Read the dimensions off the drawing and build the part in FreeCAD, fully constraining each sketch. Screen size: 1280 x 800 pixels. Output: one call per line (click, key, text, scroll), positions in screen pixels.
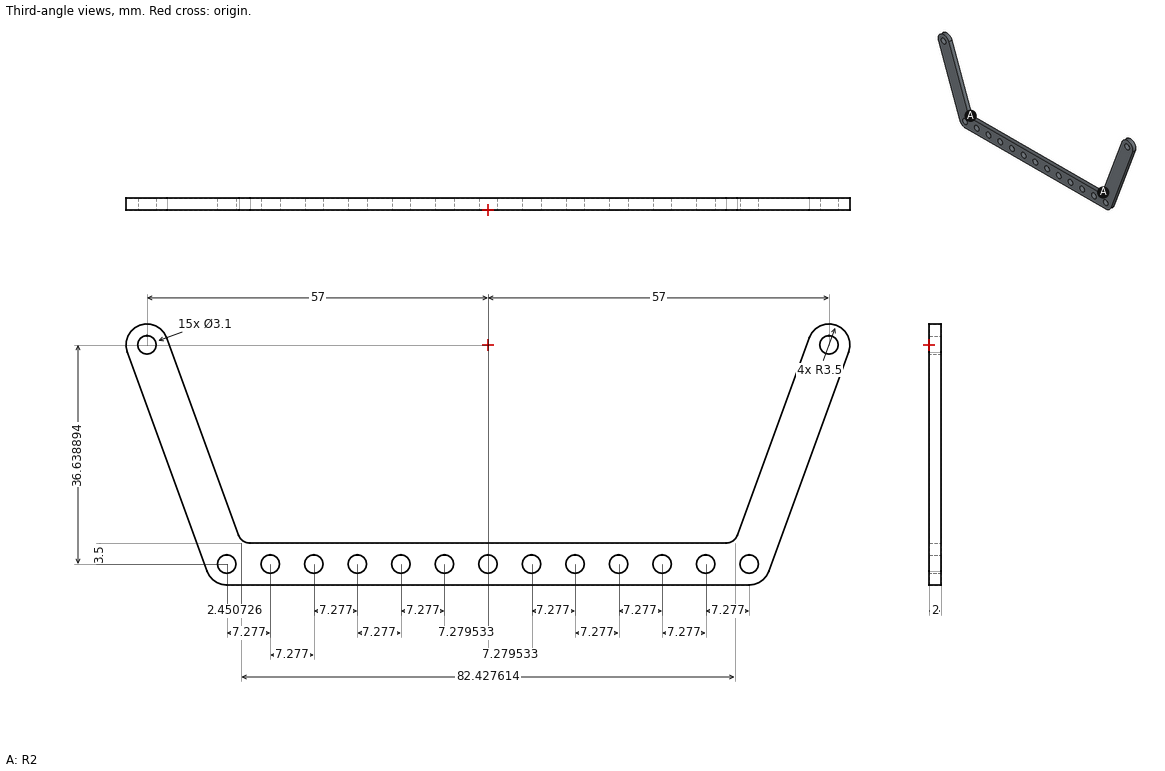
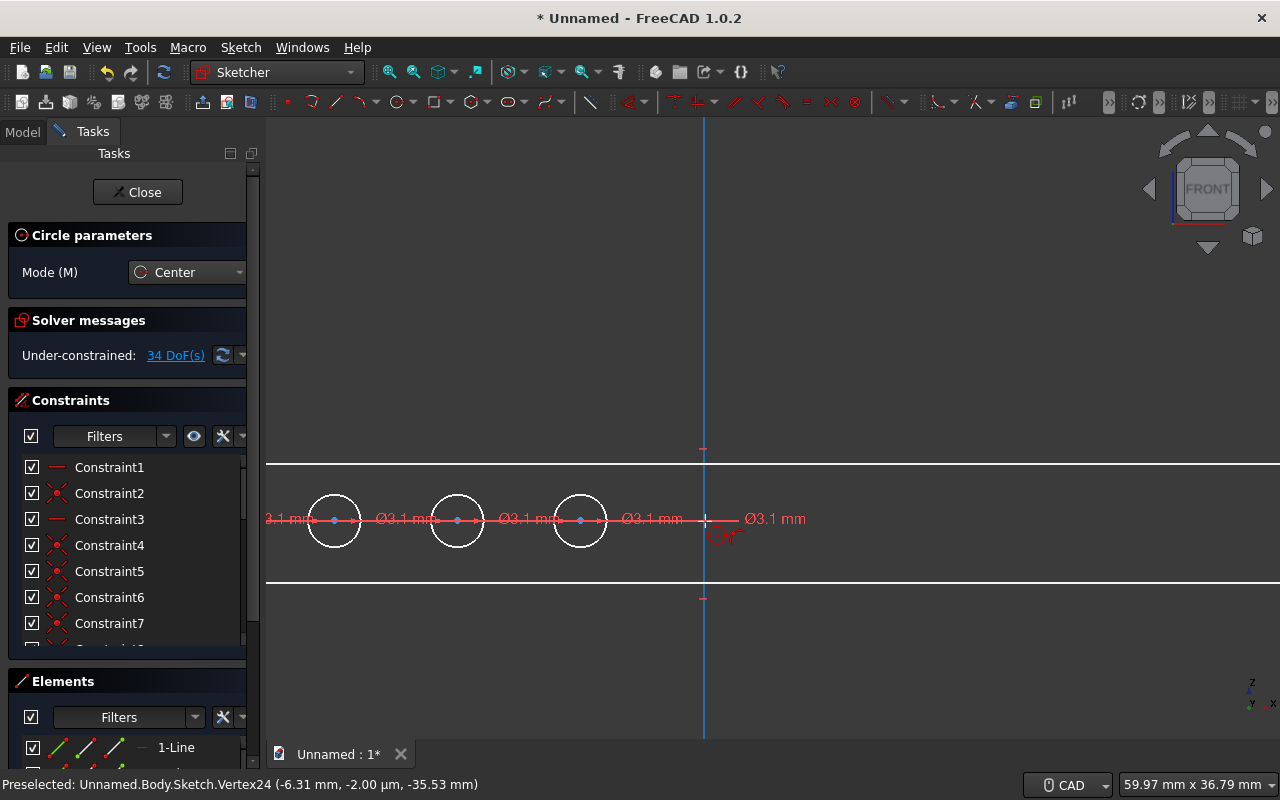
click(704, 520)
move(722, 501)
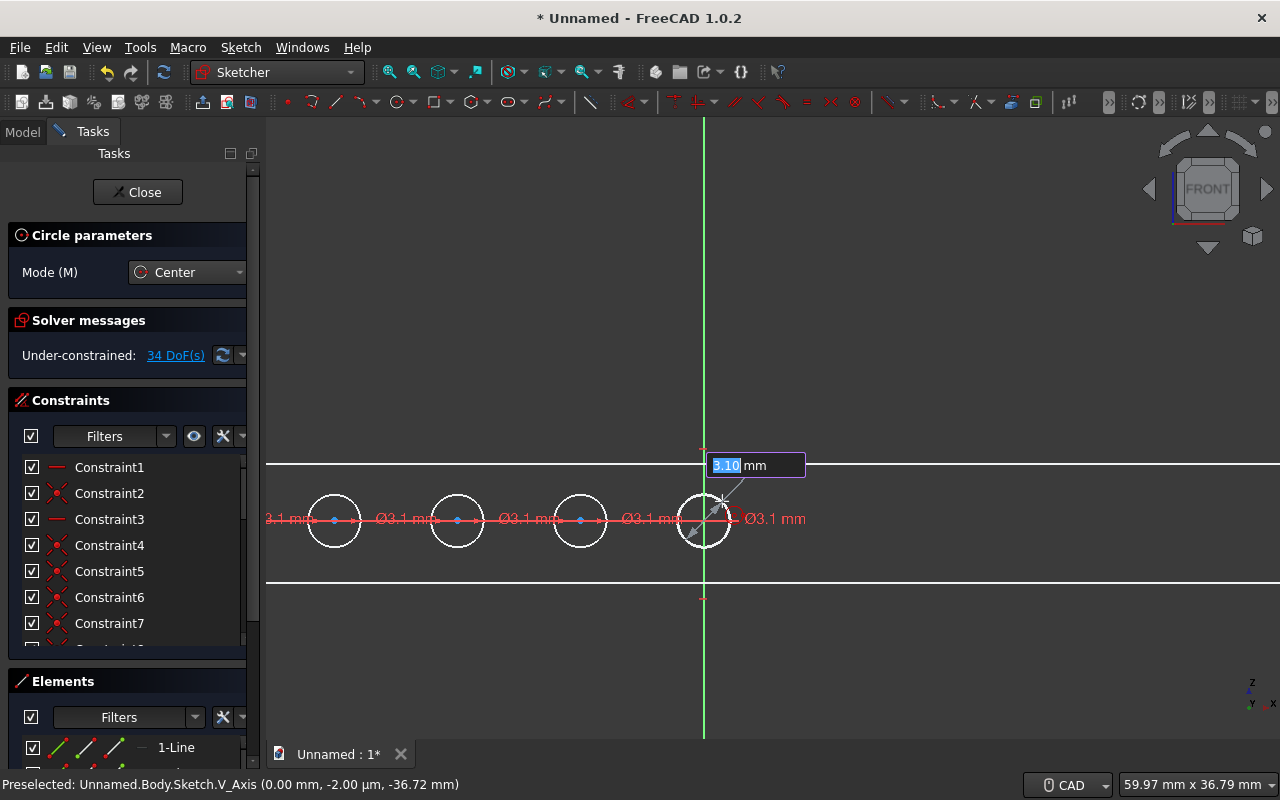
text(3.1)
key(Return)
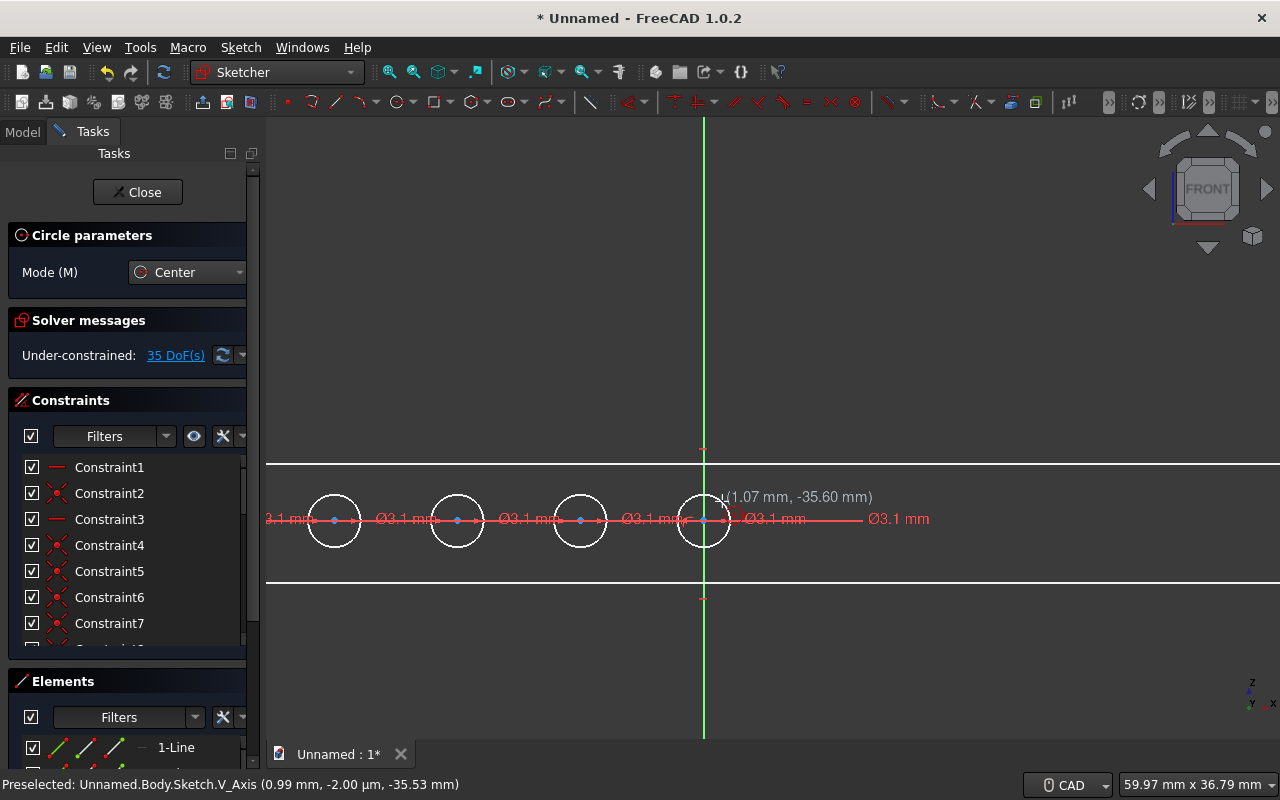
click(827, 520)
move(846, 501)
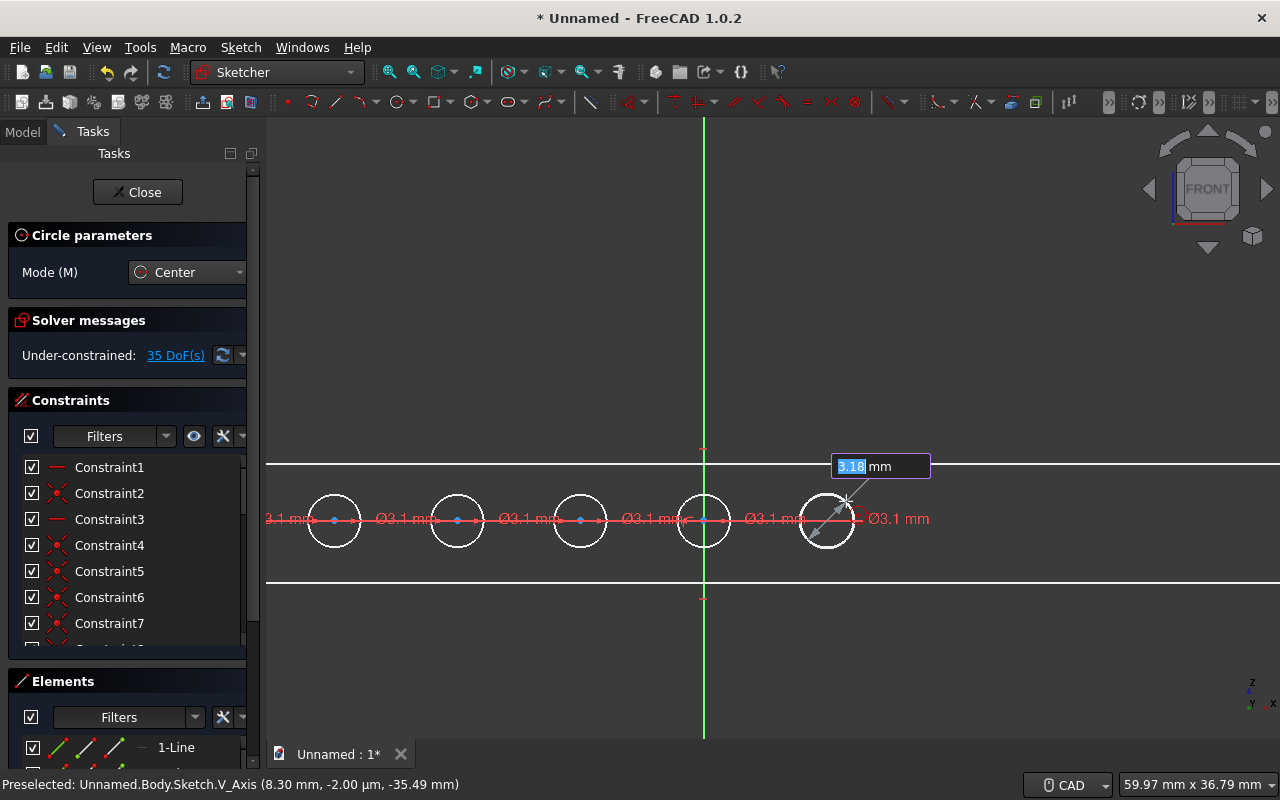
text(3.1)
key(Return)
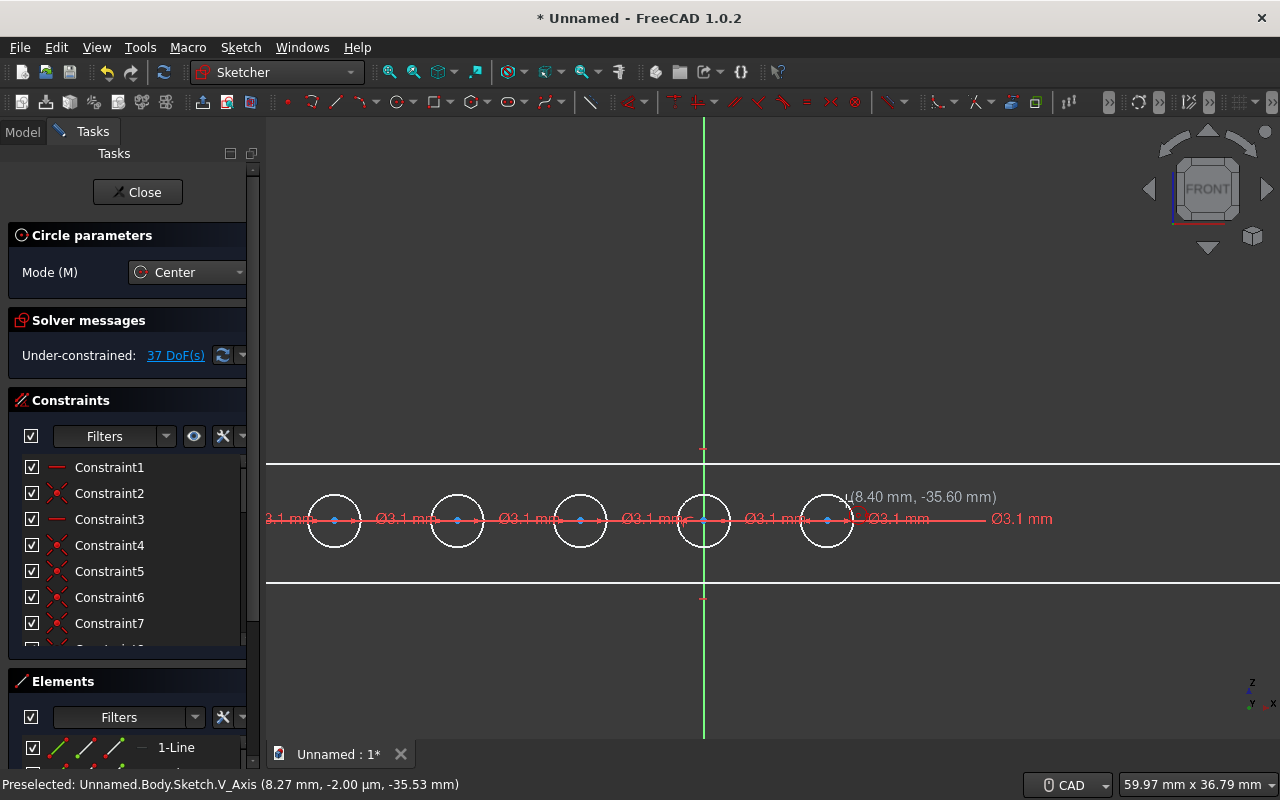
click(950, 520)
move(969, 501)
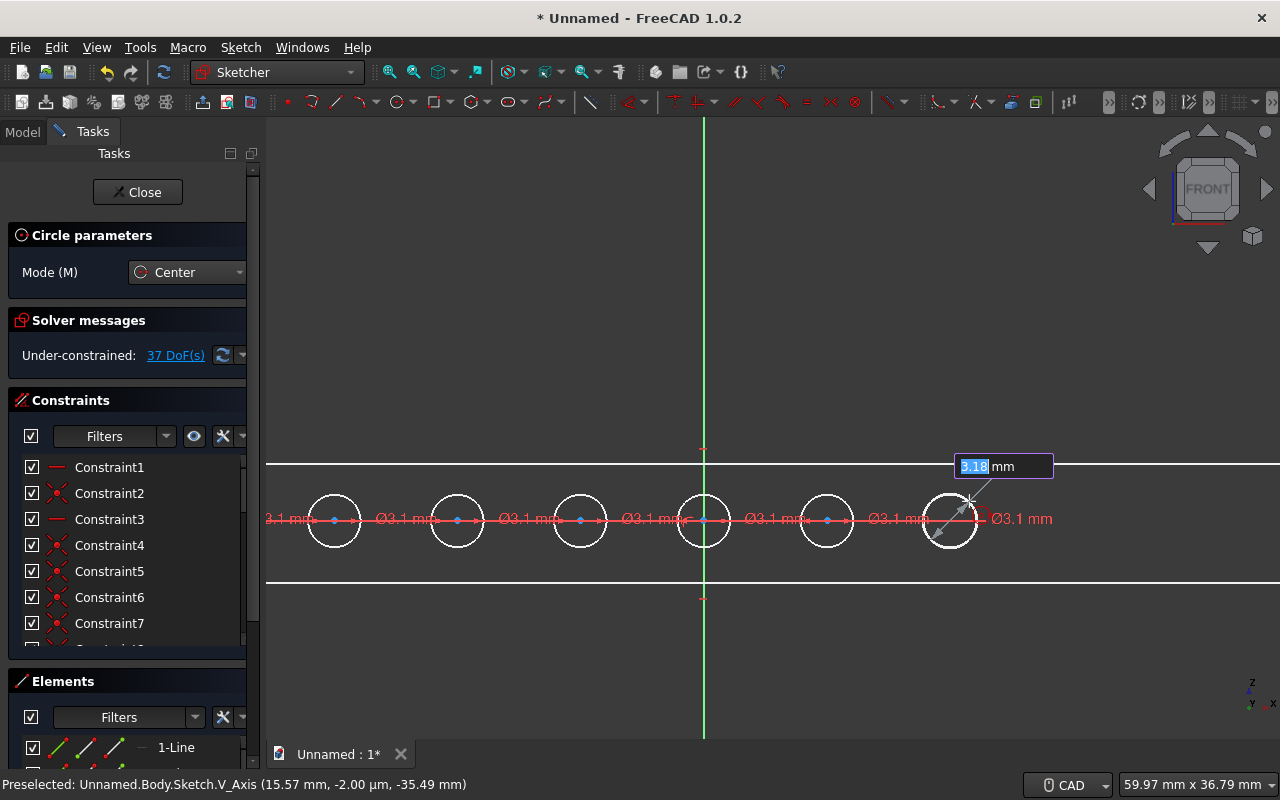
text(3.1)
key(Return)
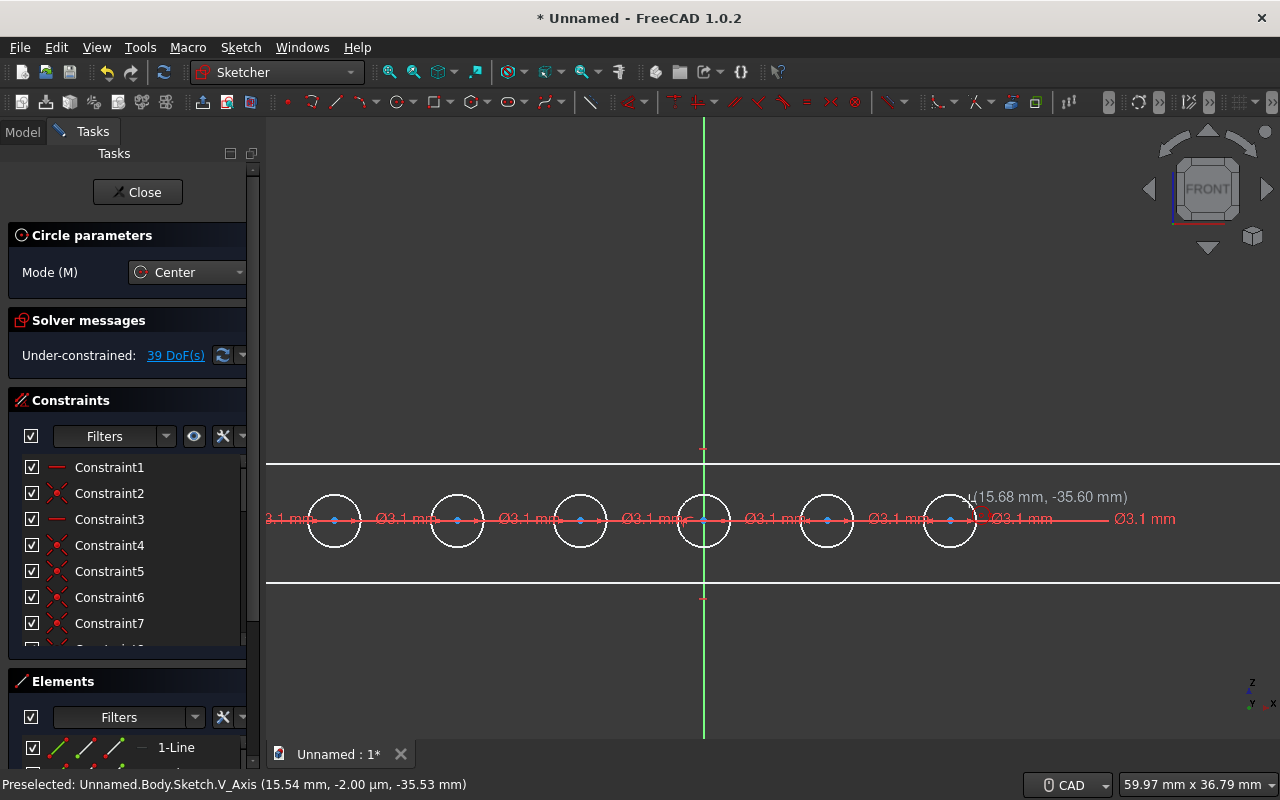
click(1073, 520)
move(1092, 501)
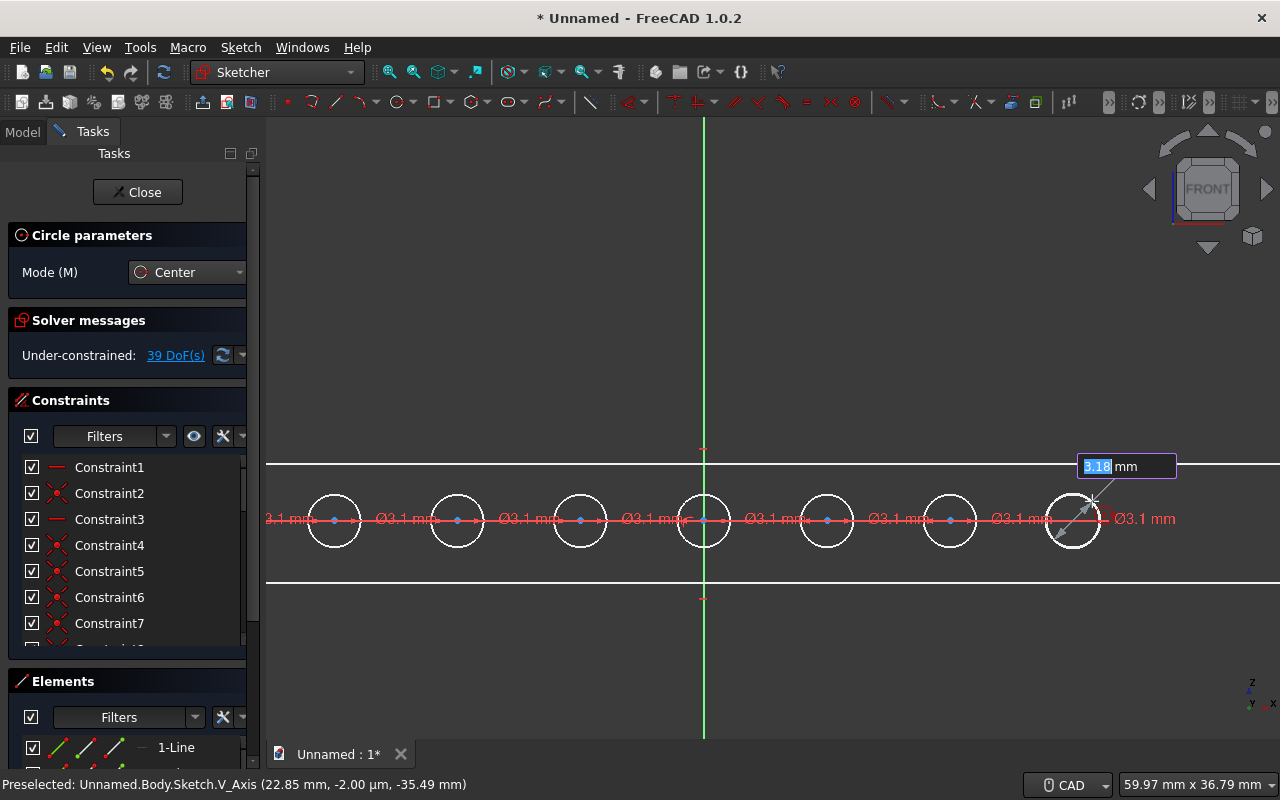
text(3.1)
key(Return)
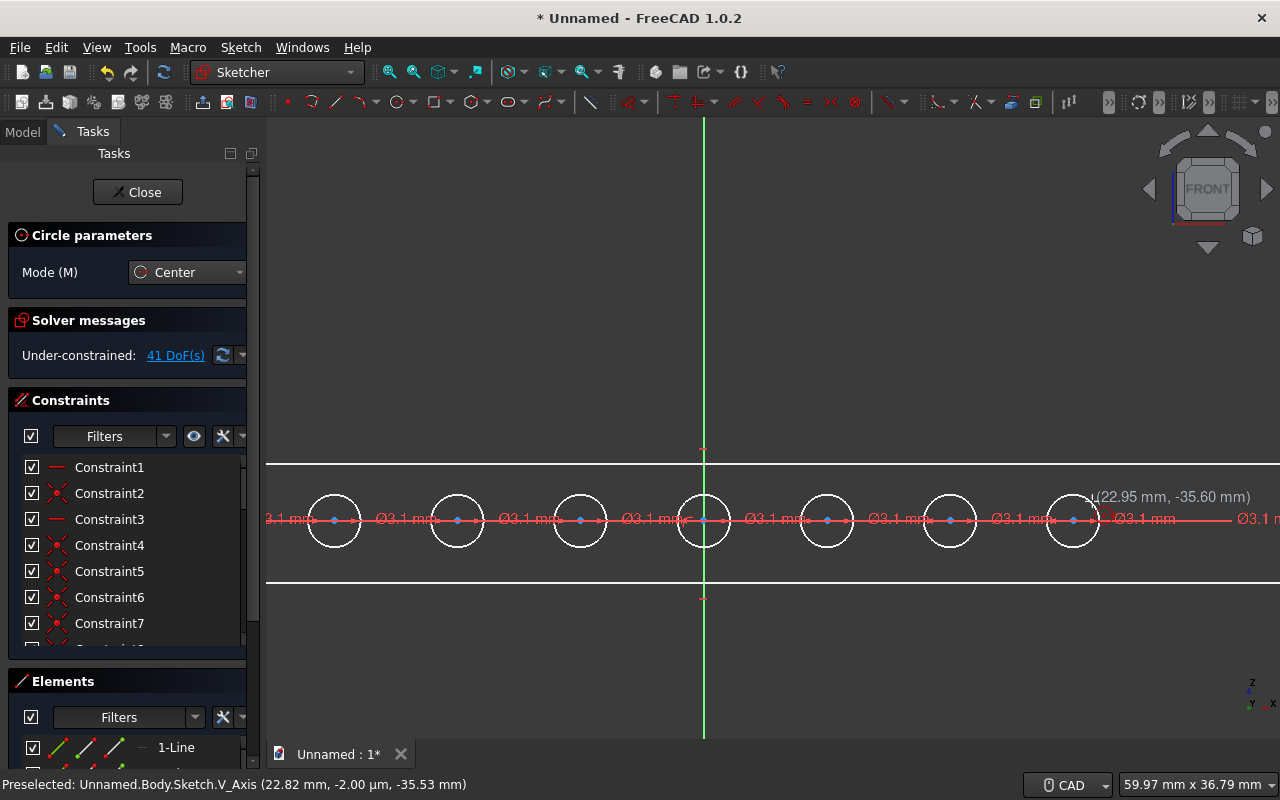
scroll(705, 521, down, 6)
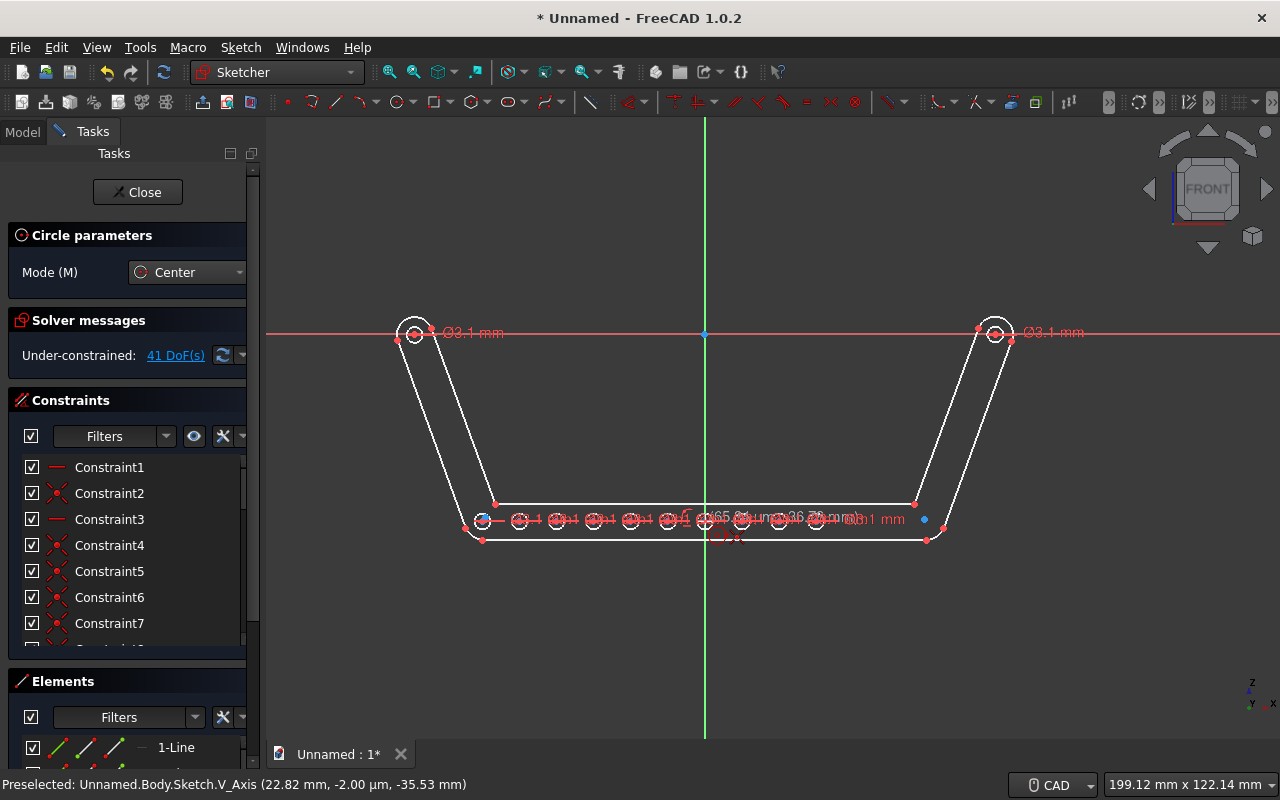
scroll(853, 521, up, 6)